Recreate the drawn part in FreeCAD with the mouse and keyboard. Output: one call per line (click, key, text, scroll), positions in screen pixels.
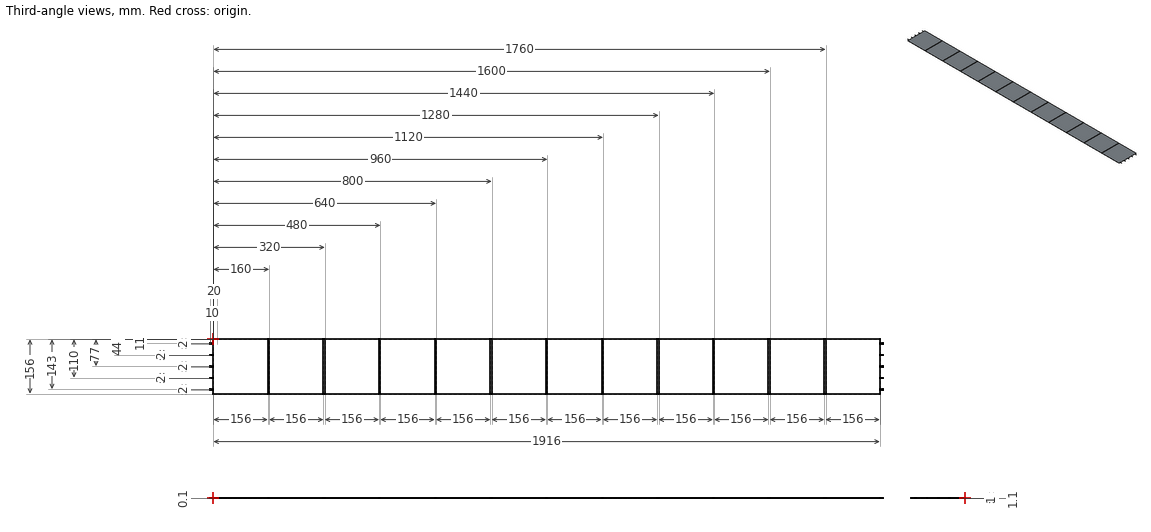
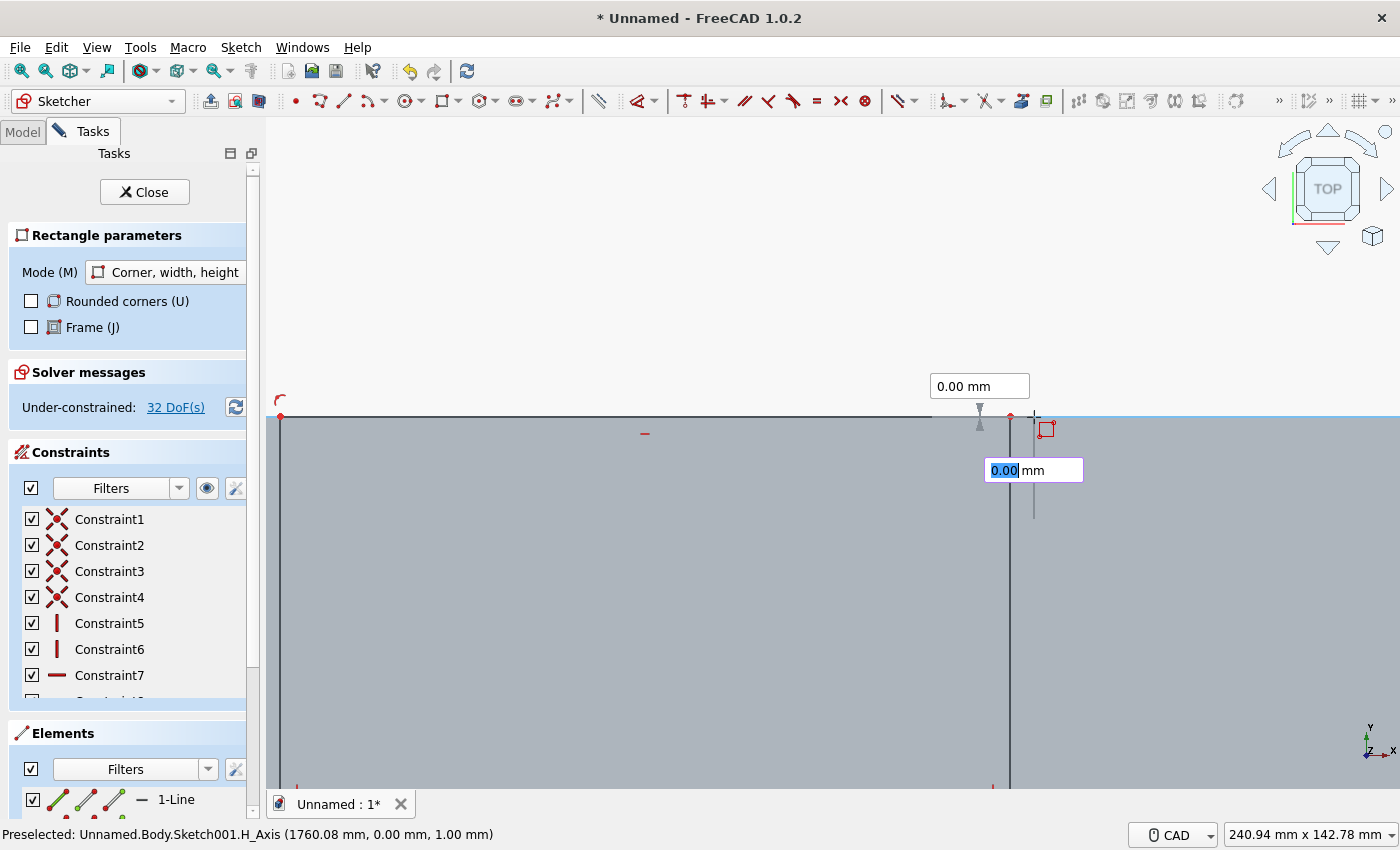
scroll(1046, 426, down, 13)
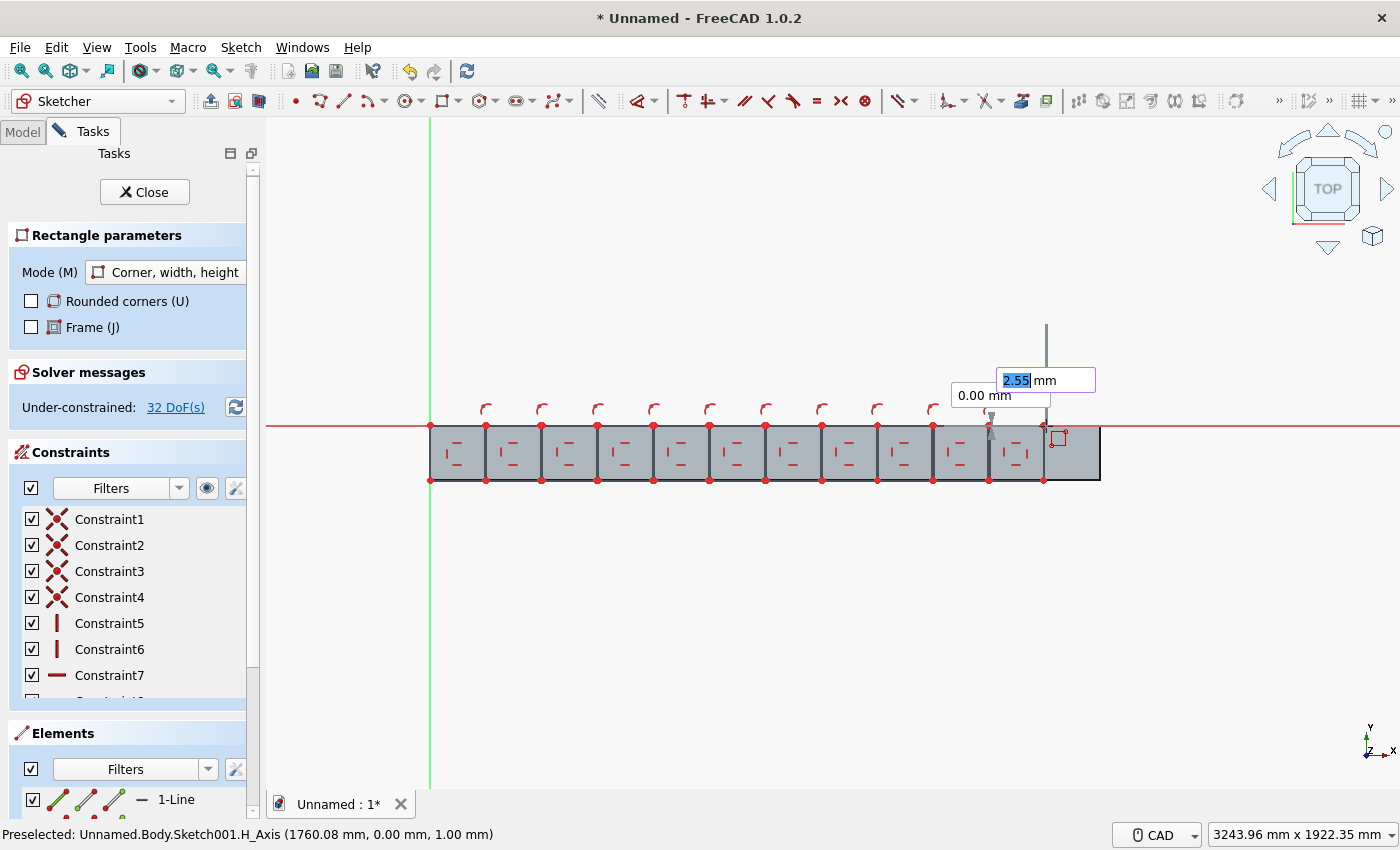
click(1100, 480)
key(Escape)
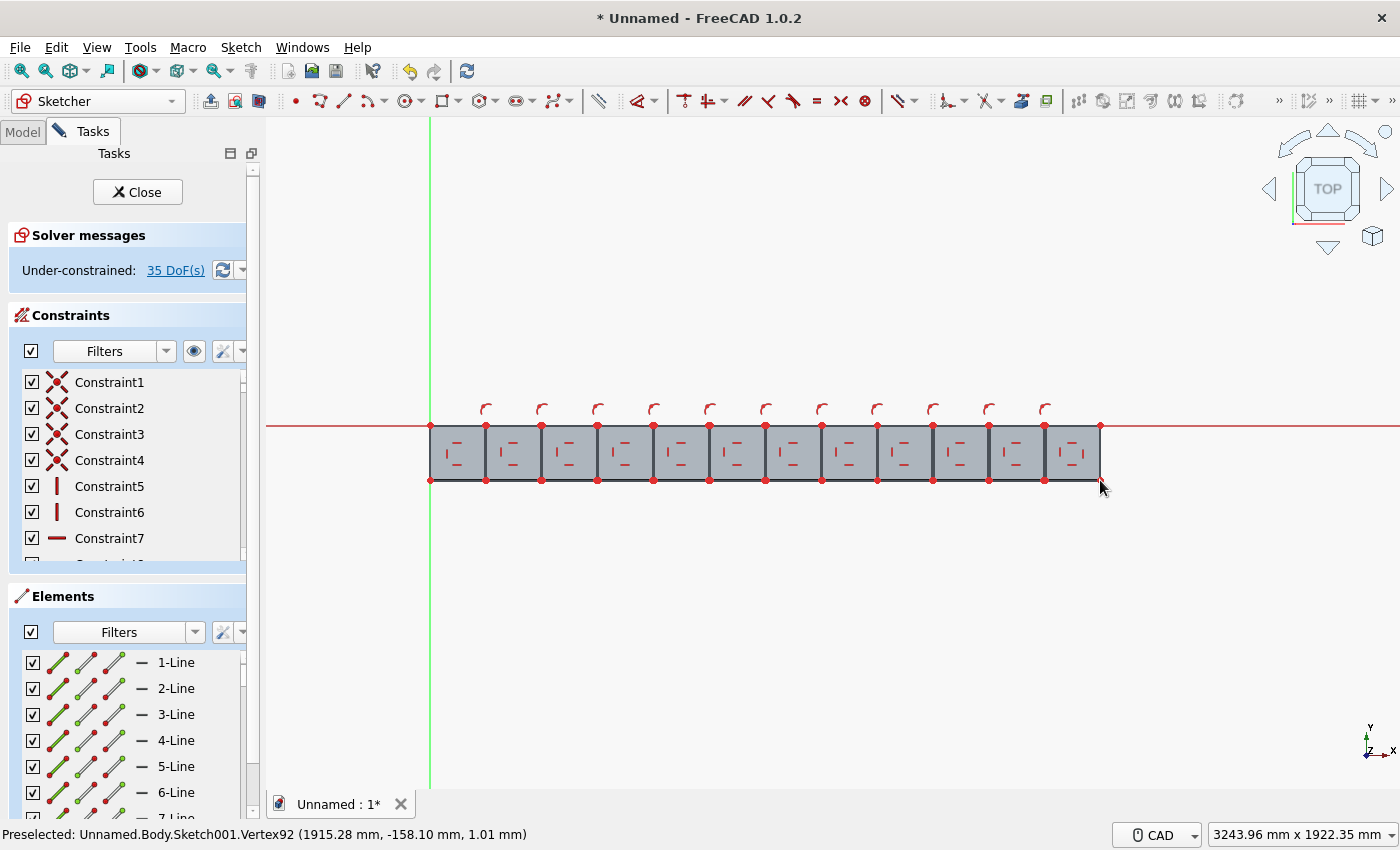
key(d)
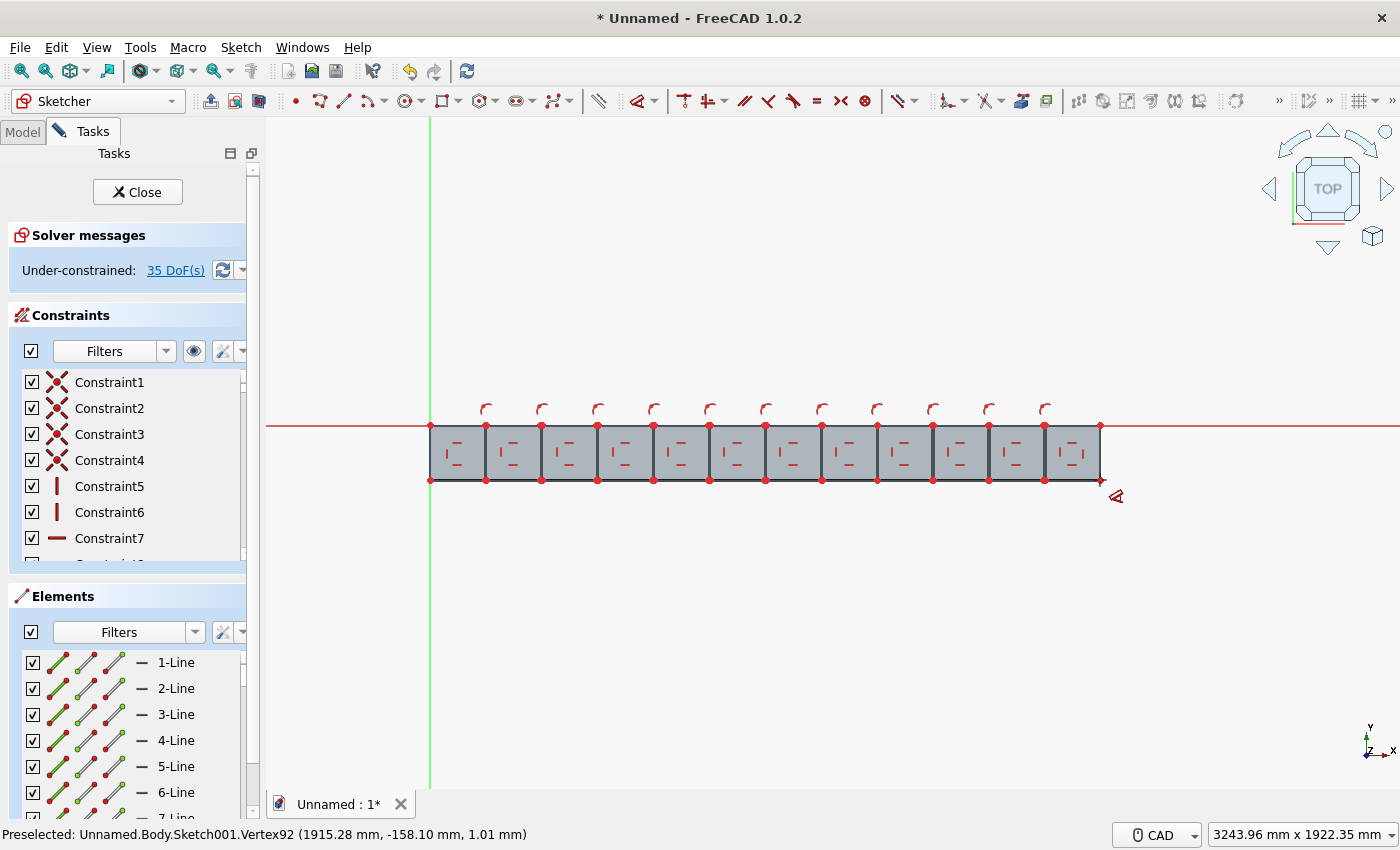
click(430, 442)
click(396, 453)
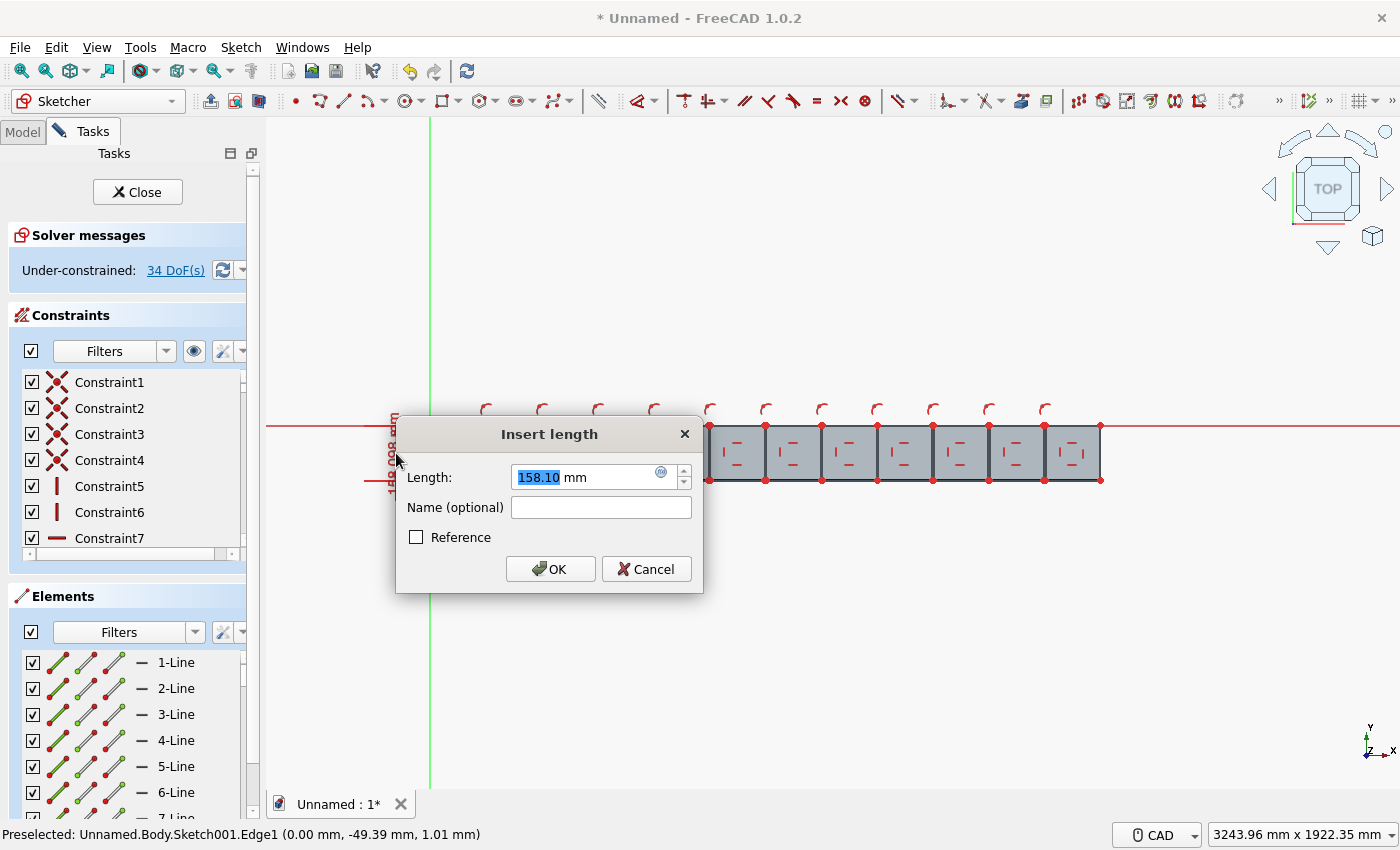
text(156)
key(Return)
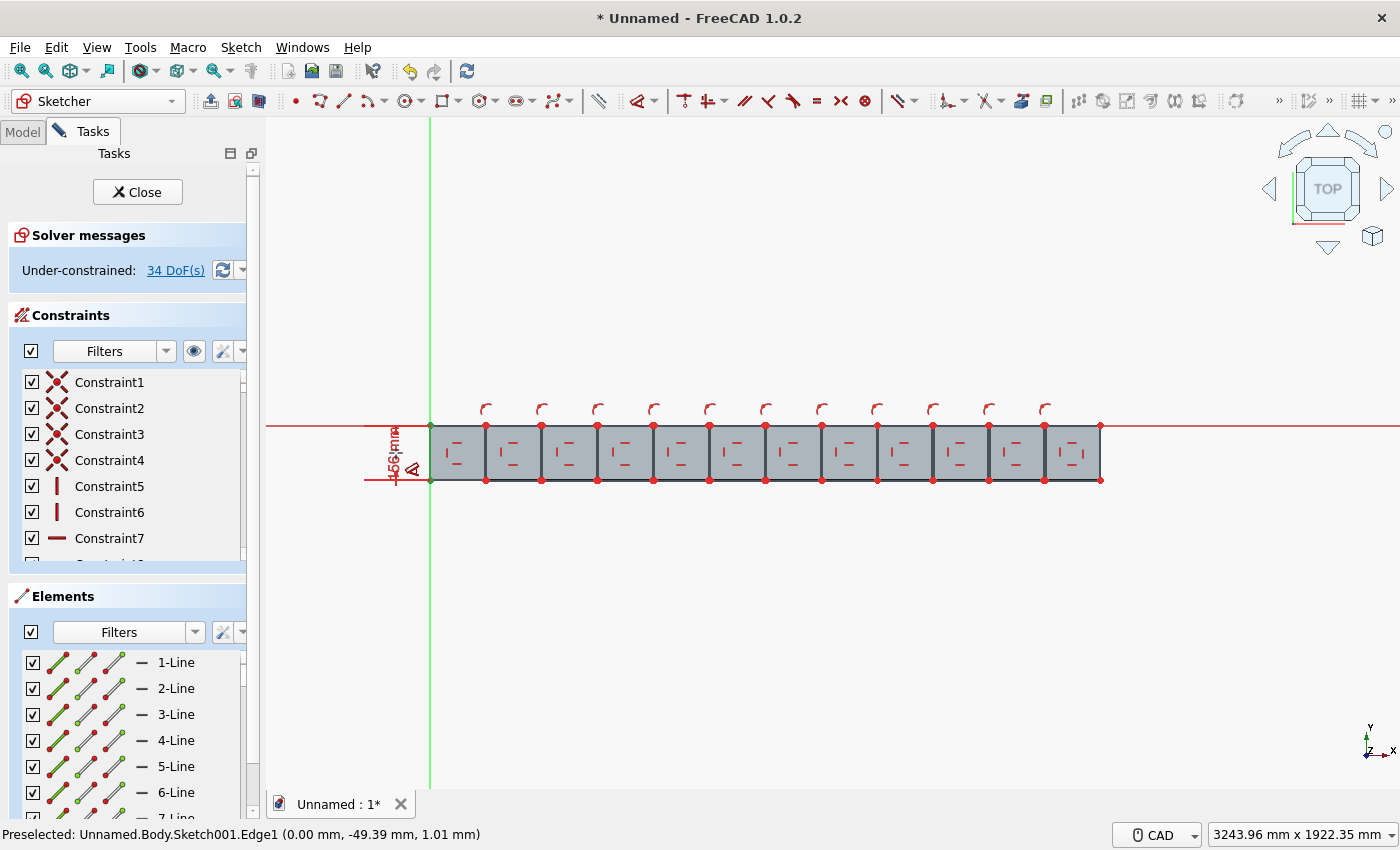
click(447, 480)
click(458, 514)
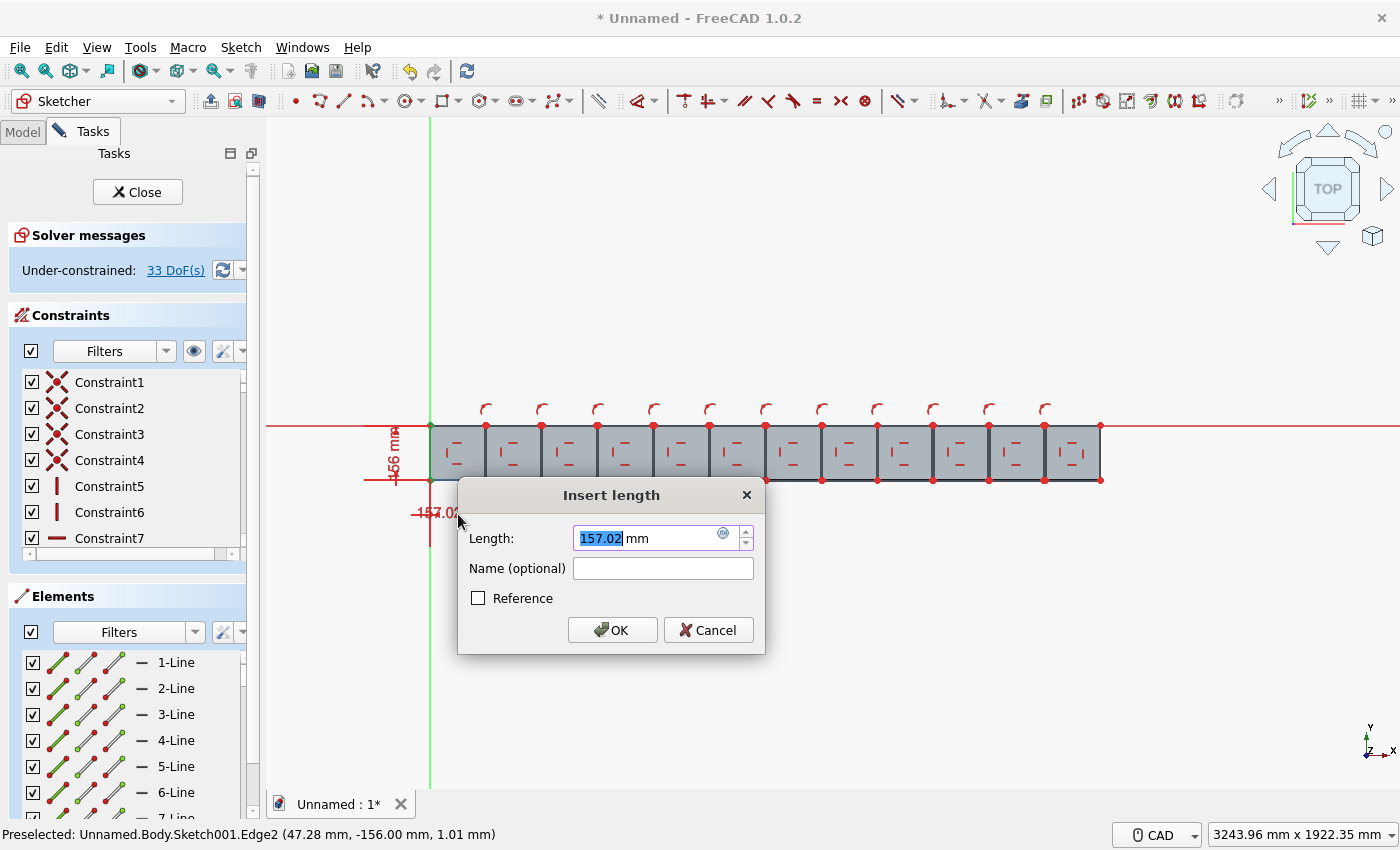
text(156)
key(Return)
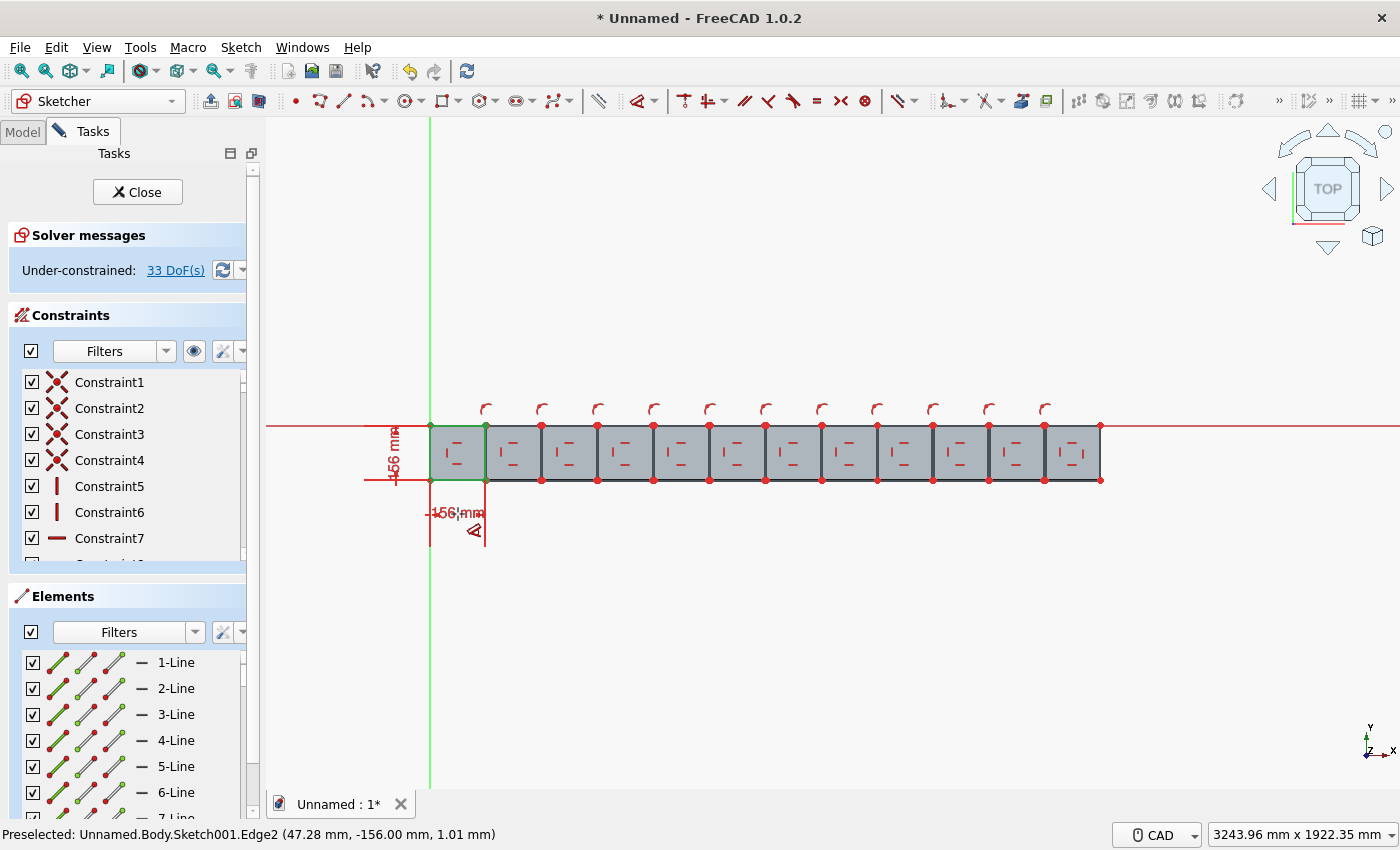
scroll(486, 442, up, 12)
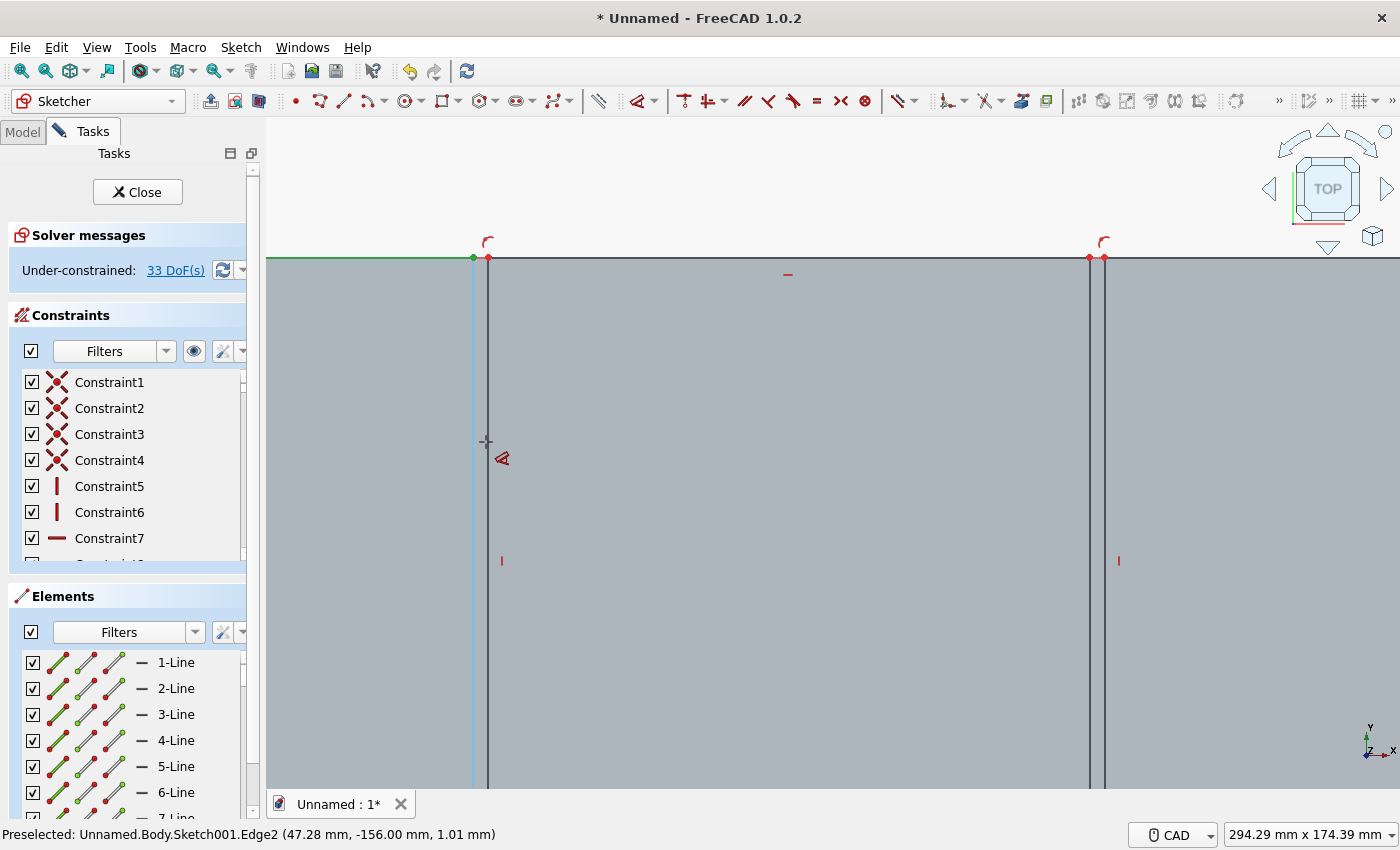
click(488, 441)
click(454, 509)